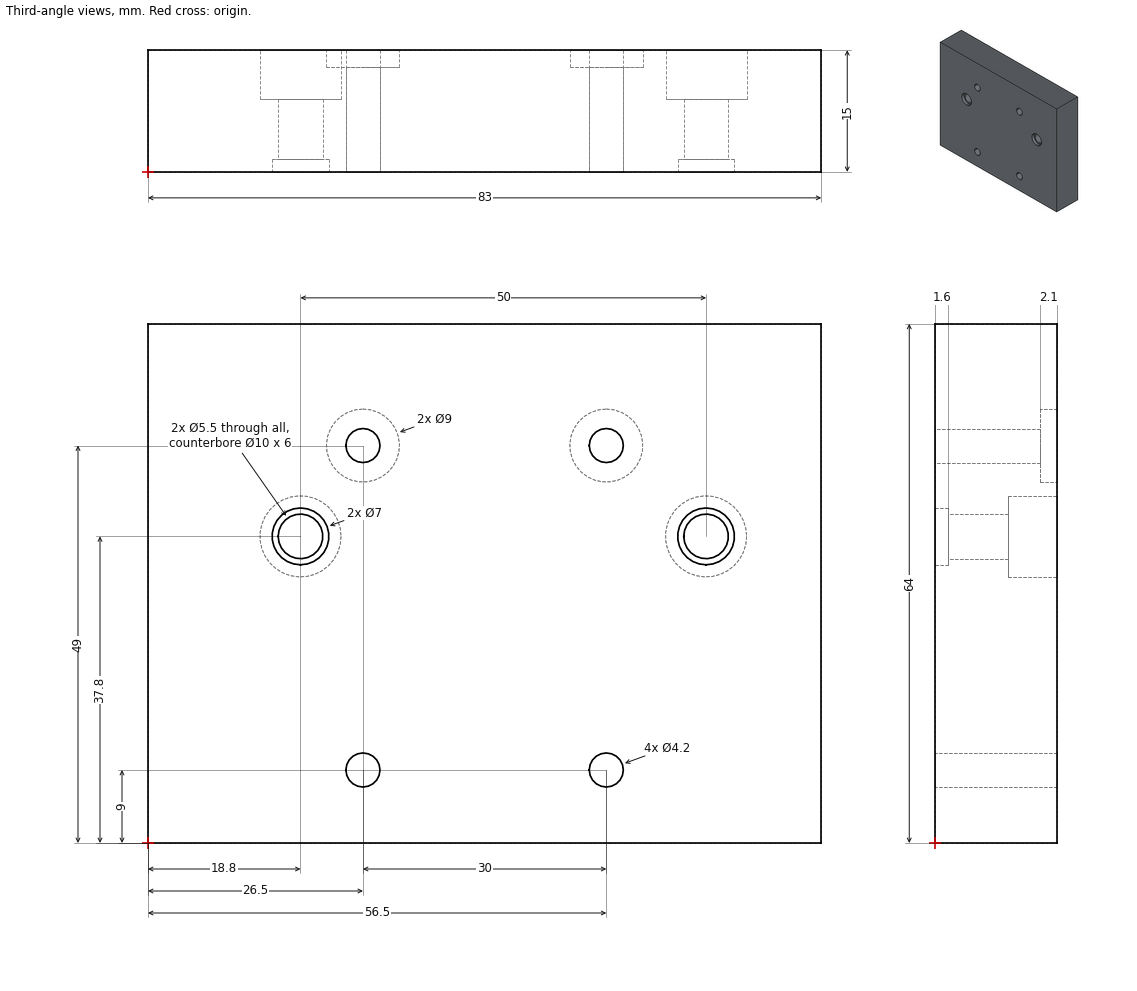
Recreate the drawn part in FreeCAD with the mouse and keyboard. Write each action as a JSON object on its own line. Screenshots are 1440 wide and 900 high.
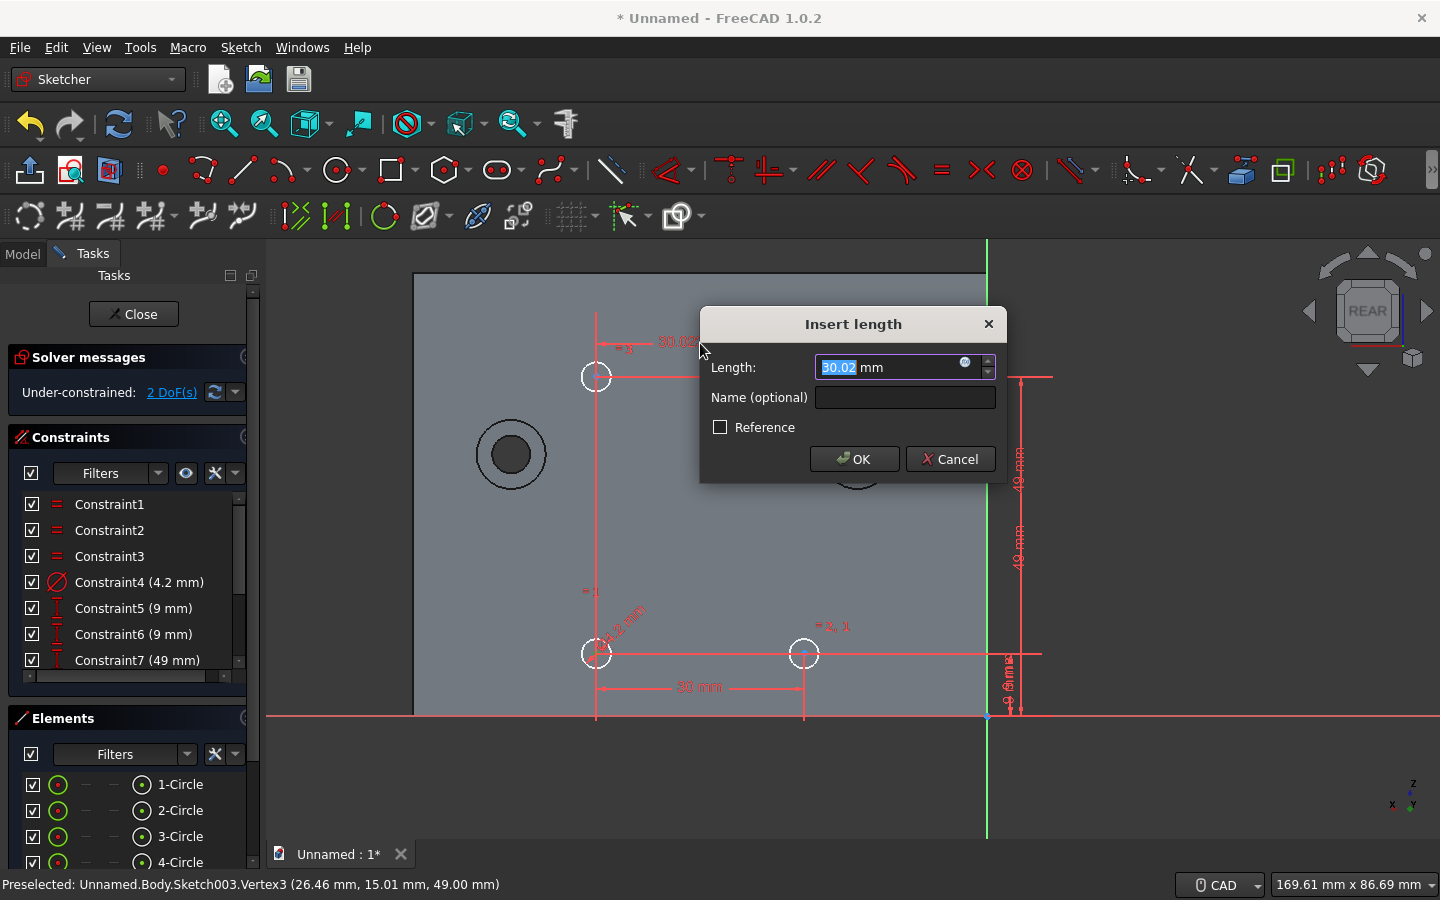
{"action": "type", "text": "30"}
{"action": "key", "text": "Return"}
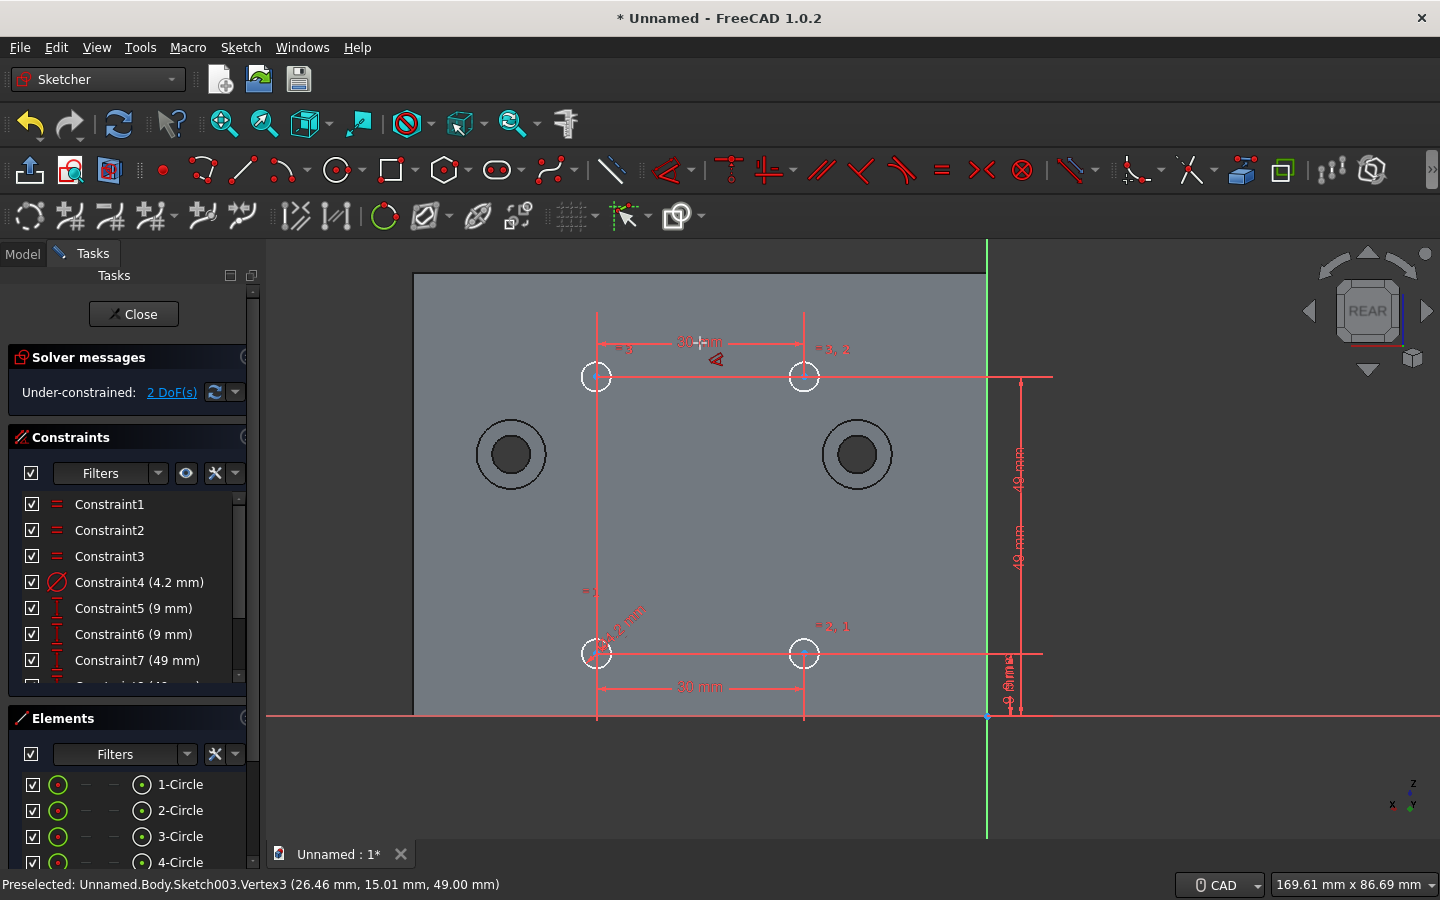
{"action": "left_click", "coordinate": [804, 377]}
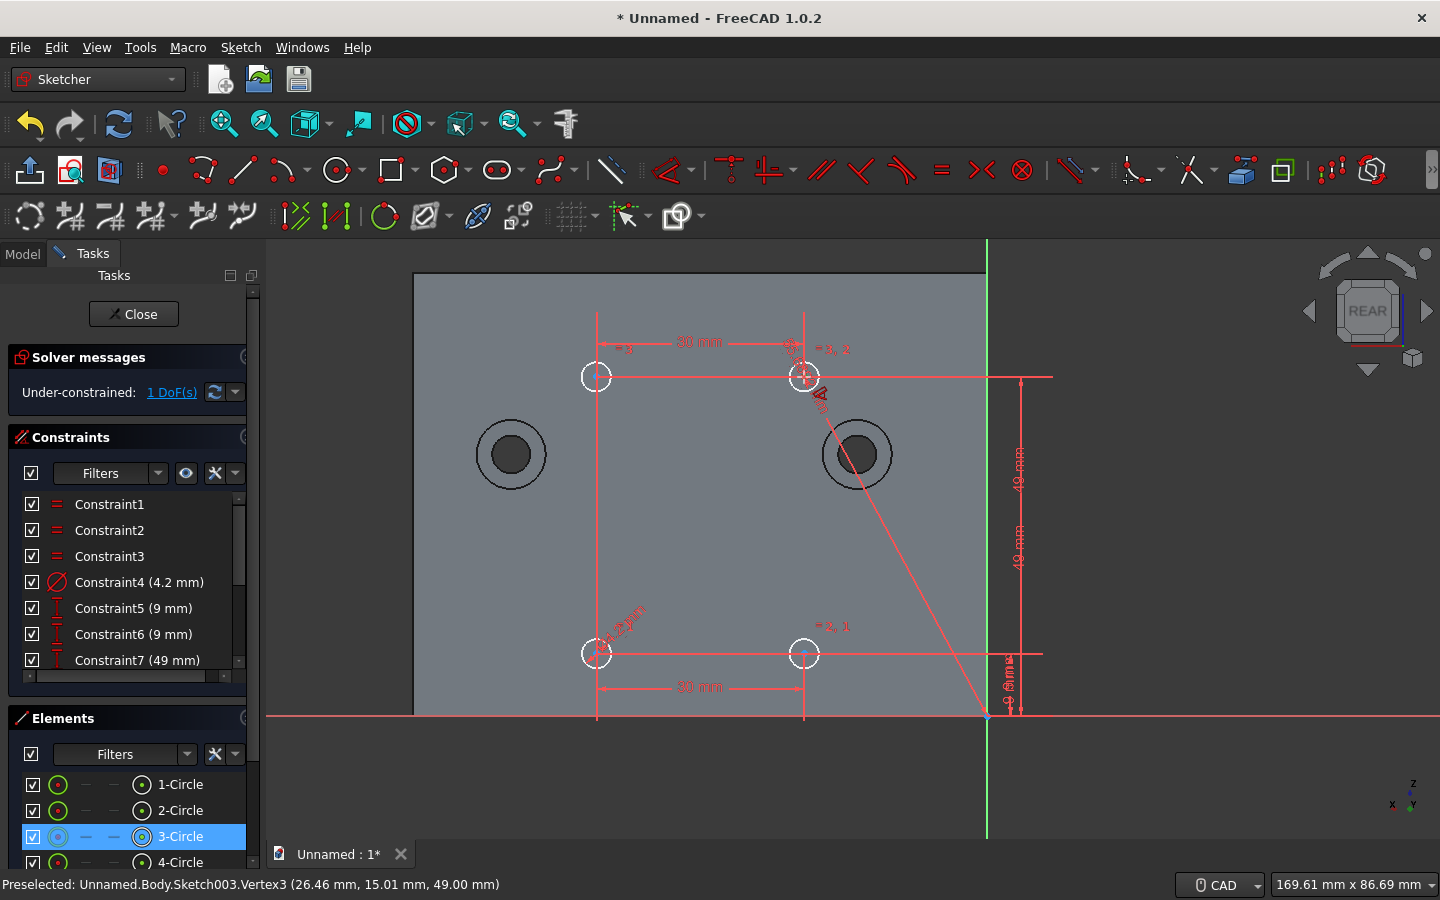
{"action": "left_click", "coordinate": [596, 377]}
{"action": "left_click", "coordinate": [627, 343]}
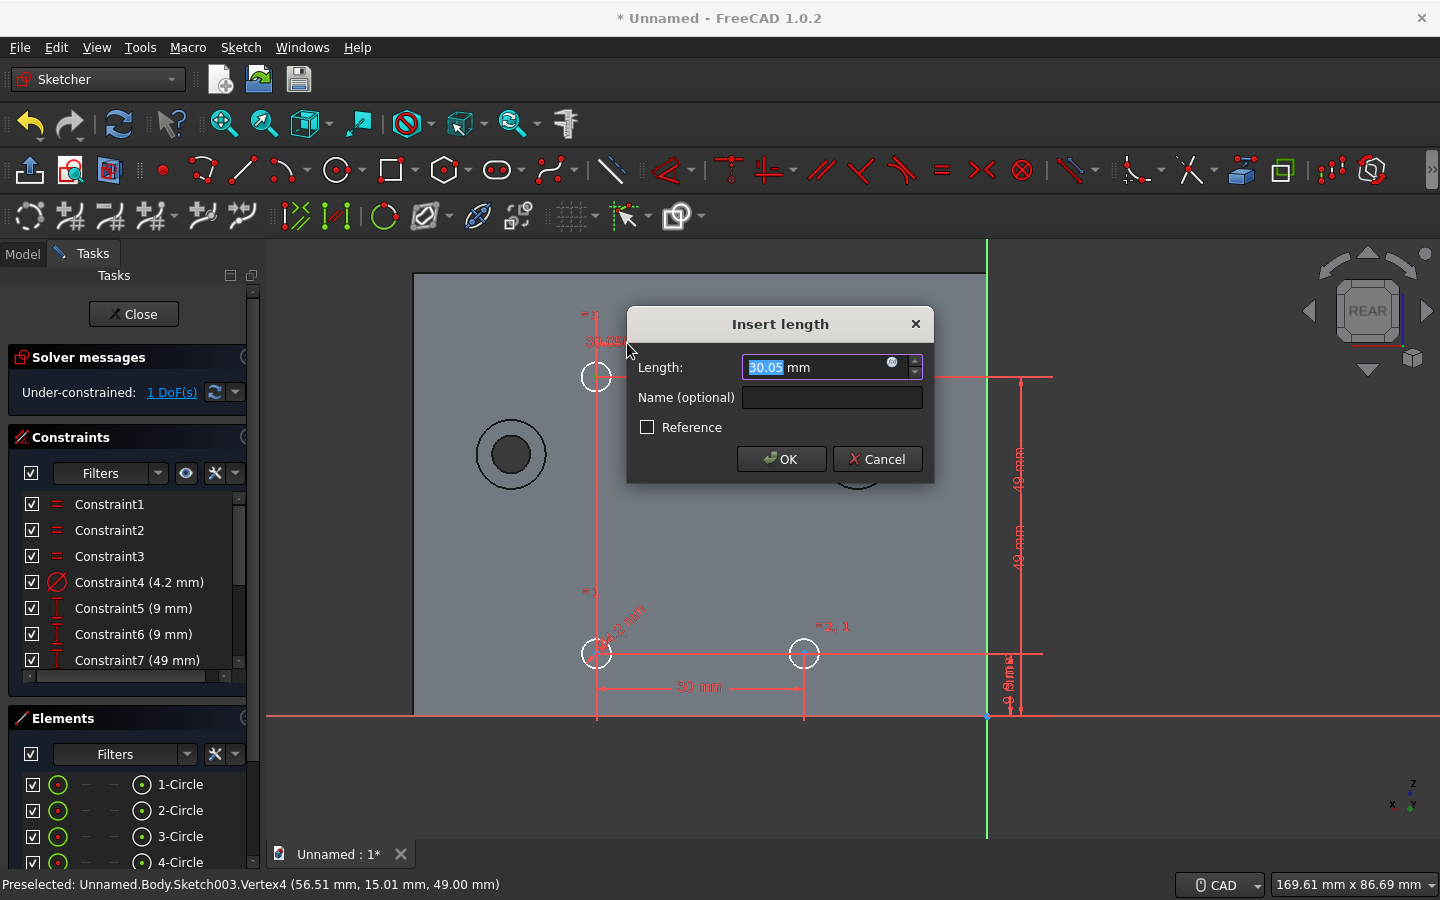
{"action": "type", "text": "30"}
{"action": "key", "text": "Return"}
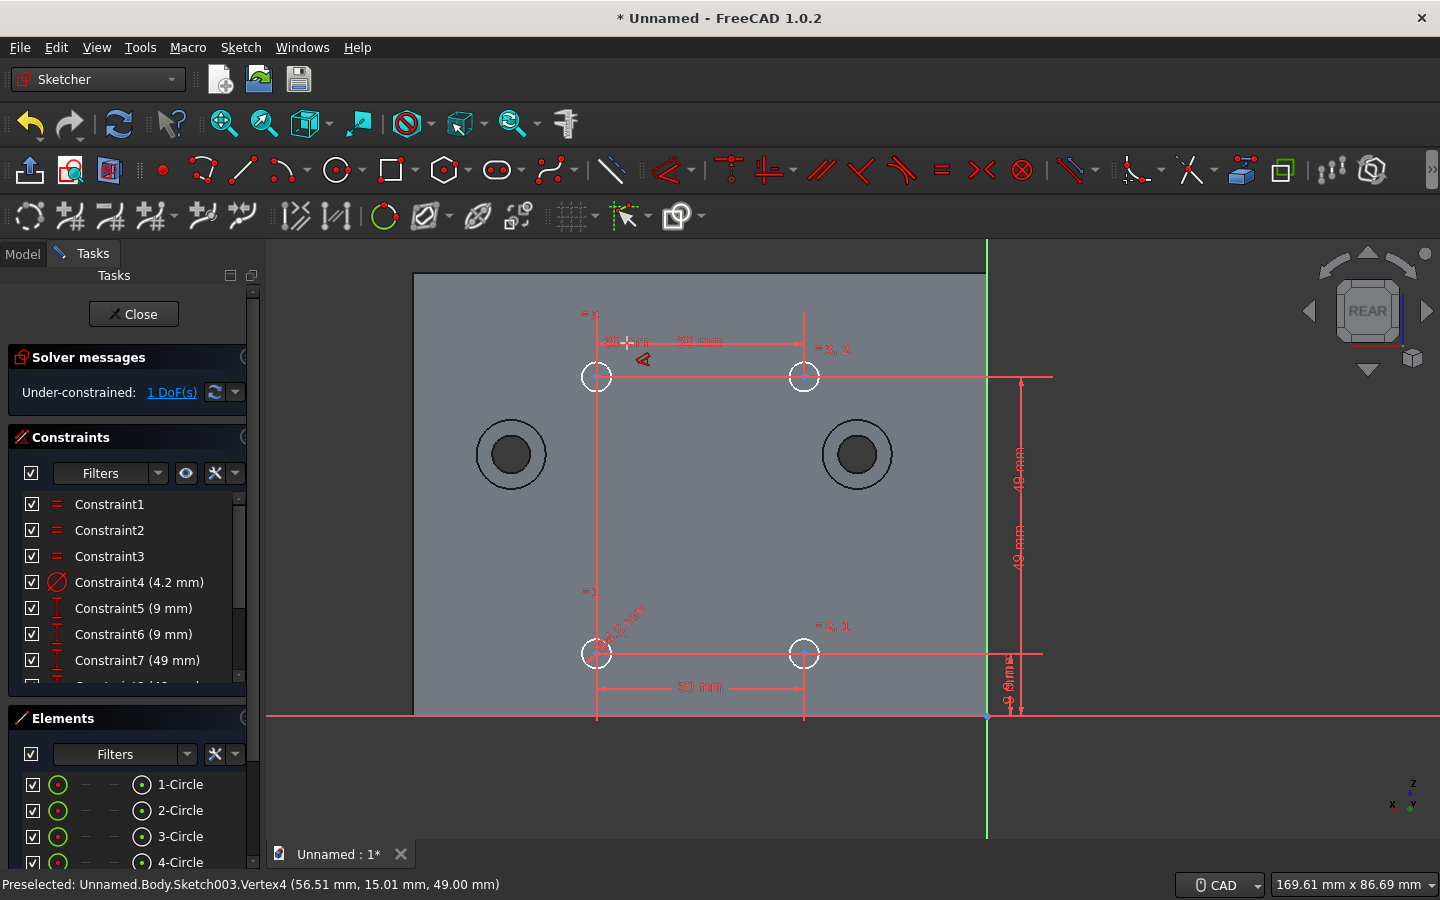
{"action": "left_click", "coordinate": [597, 654]}
{"action": "left_click", "coordinate": [792, 750]}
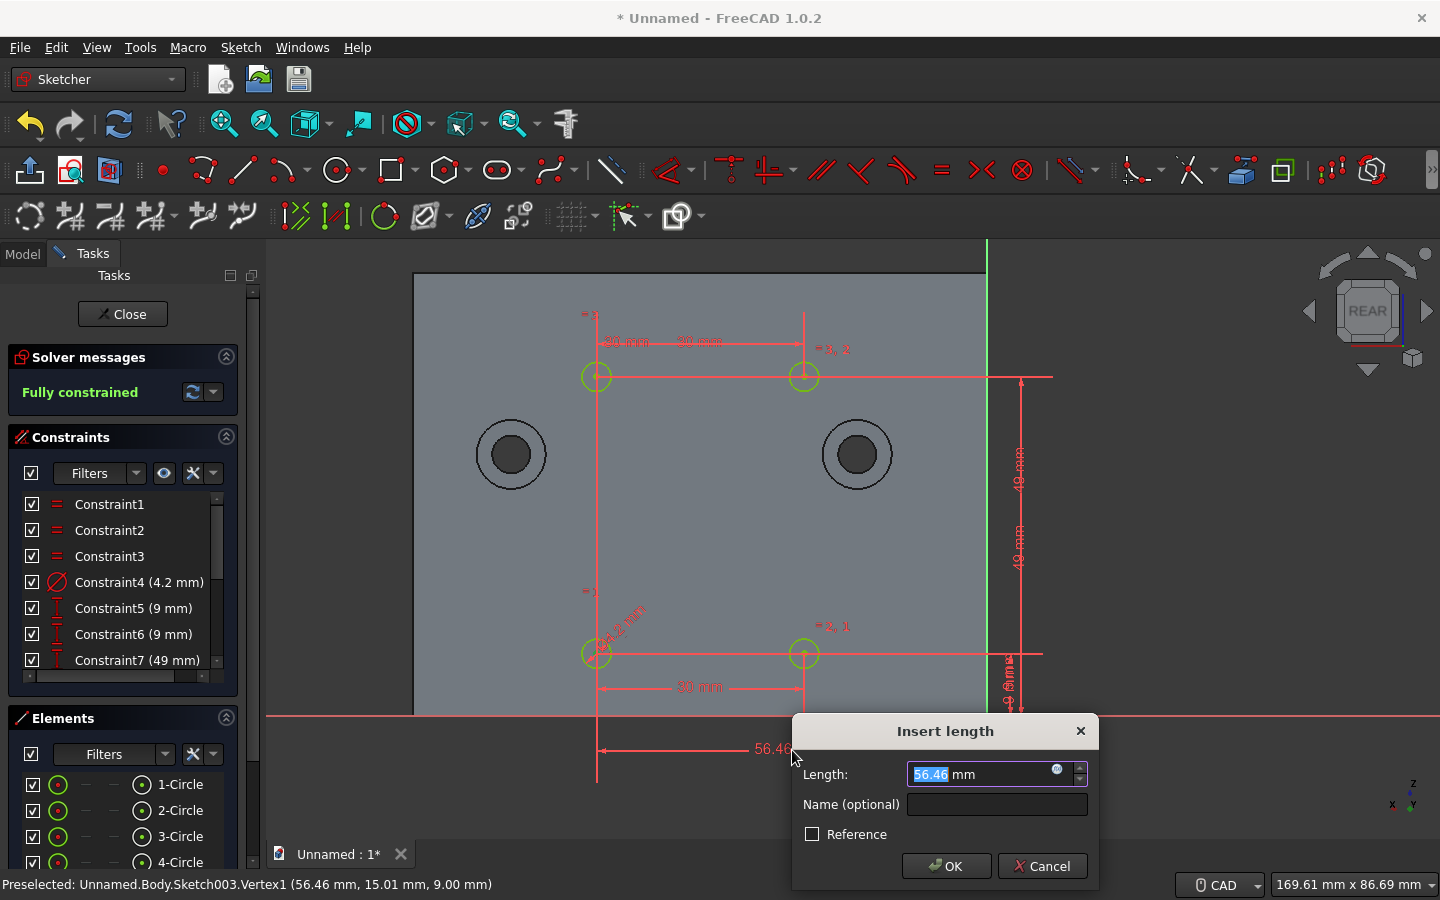
{"action": "type", "text": "56.5"}
{"action": "key", "text": "Return"}
{"action": "key", "text": "Escape"}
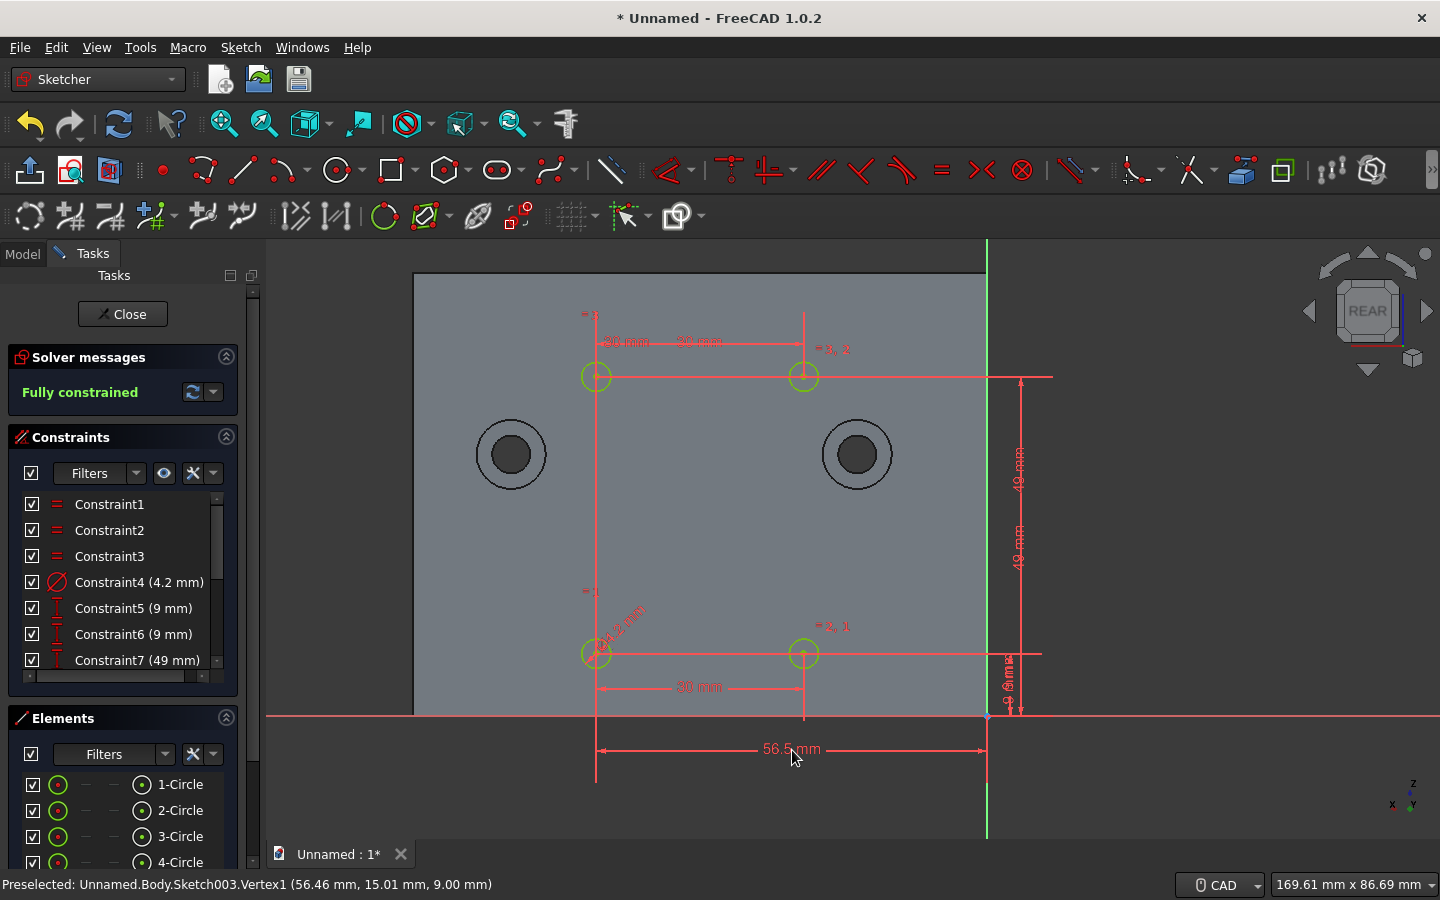
{"action": "left_click", "coordinate": [123, 314]}